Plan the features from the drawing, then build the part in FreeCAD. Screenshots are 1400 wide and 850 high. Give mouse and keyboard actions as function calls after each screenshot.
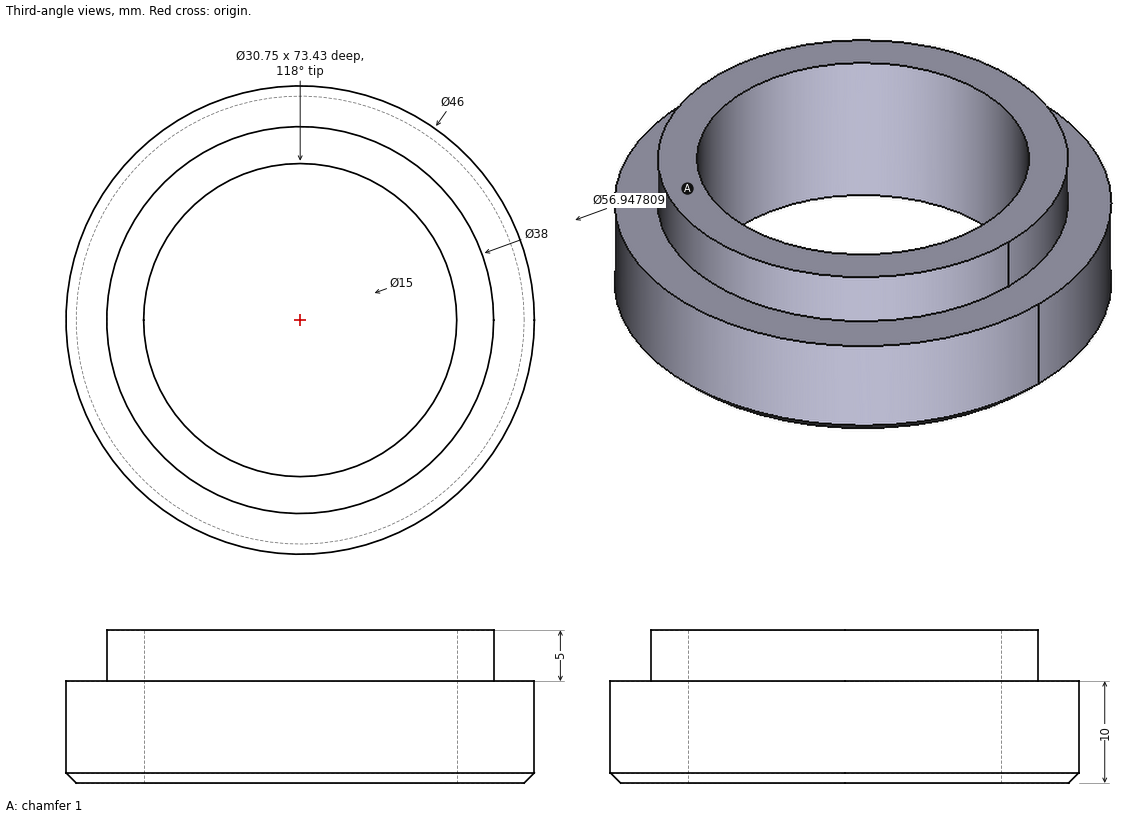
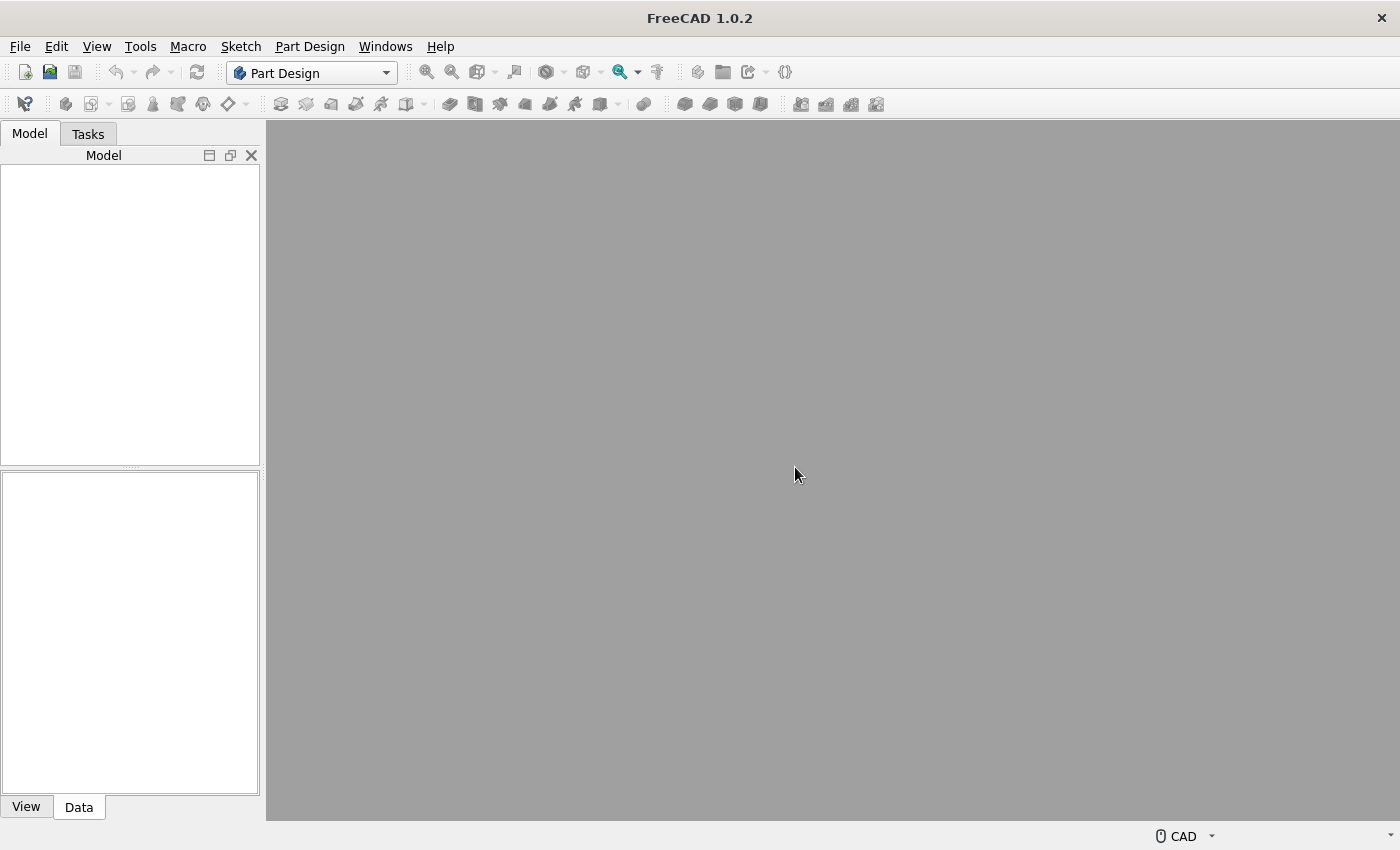
click(25, 72)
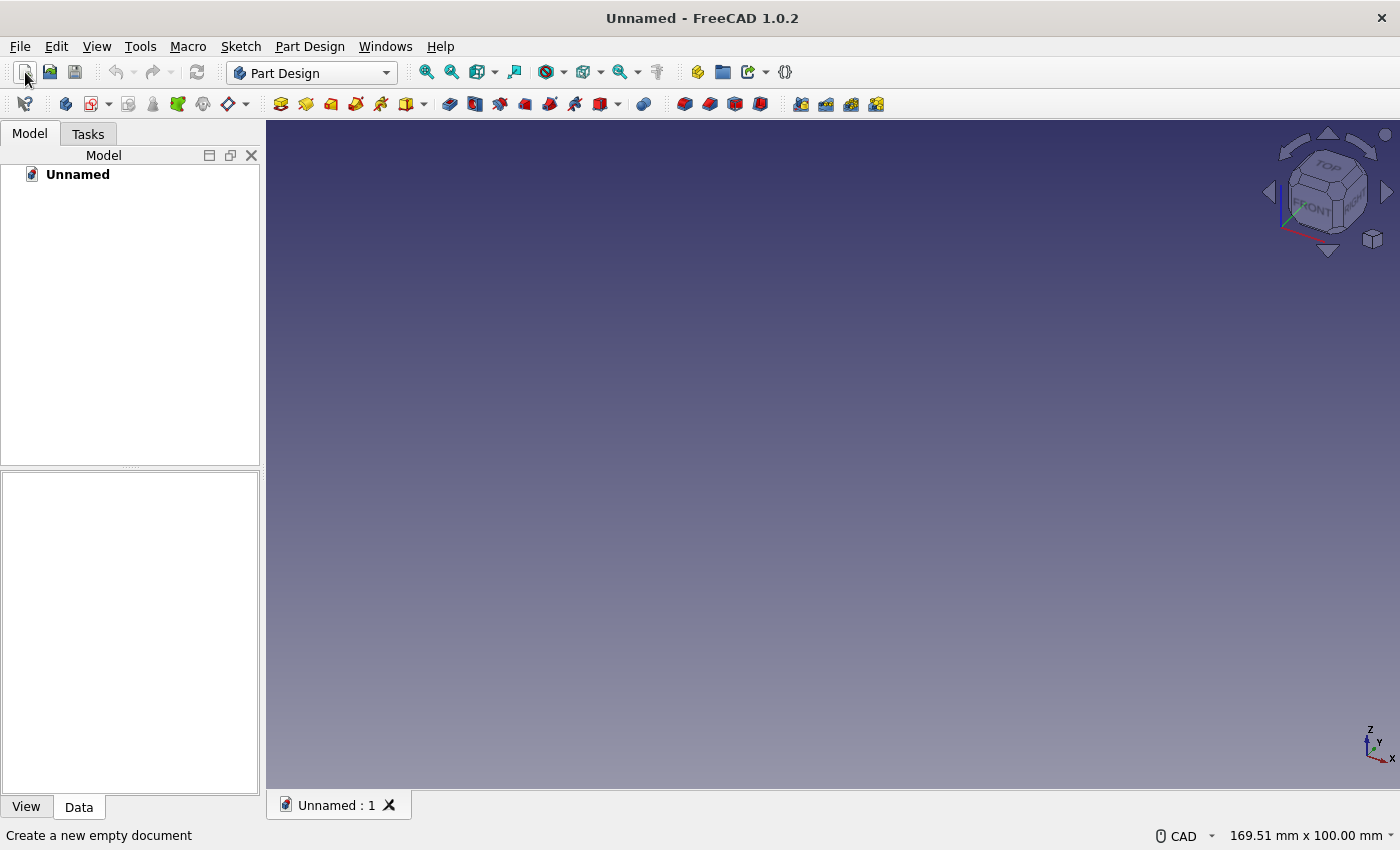
click(90, 104)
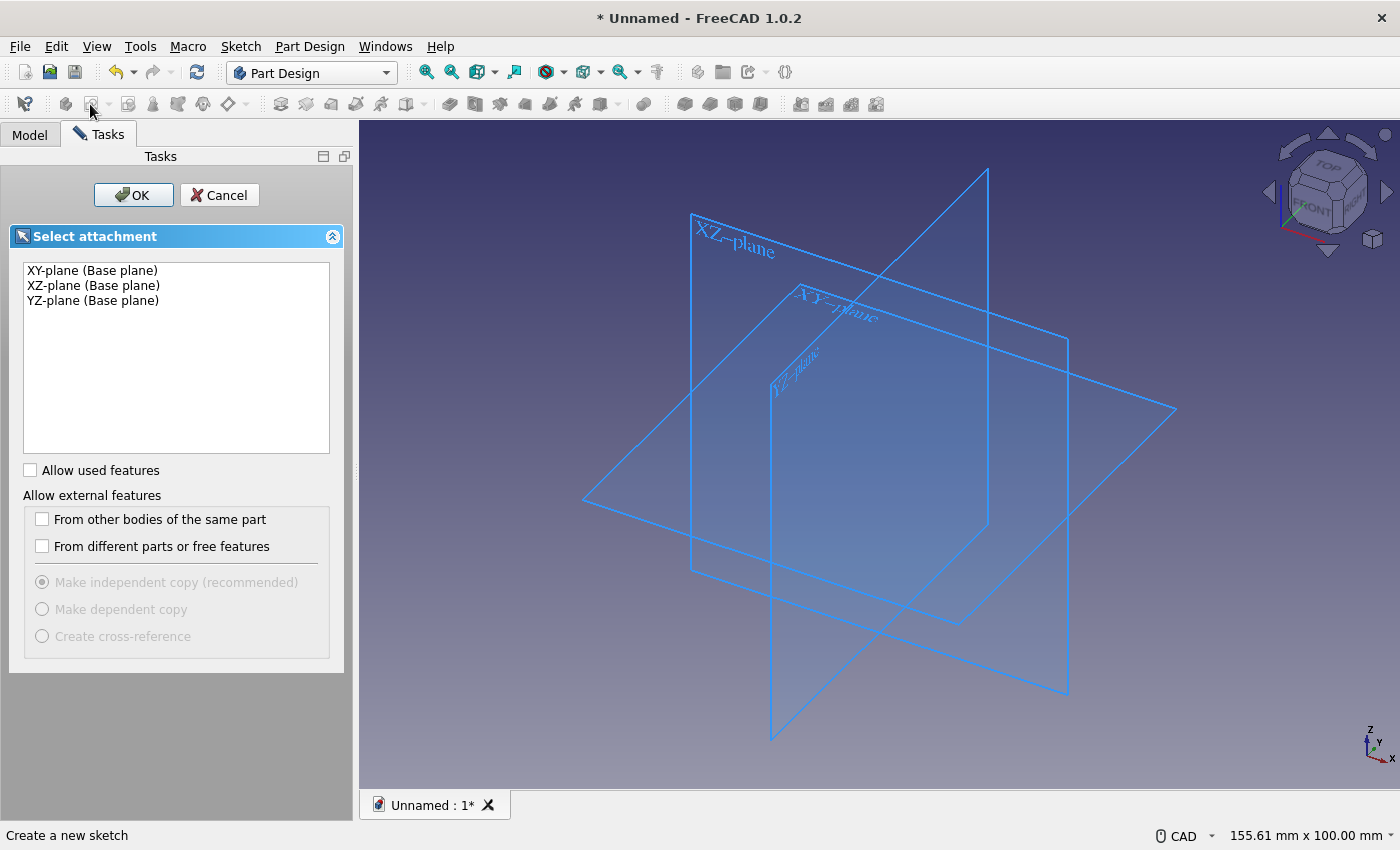
click(84, 270)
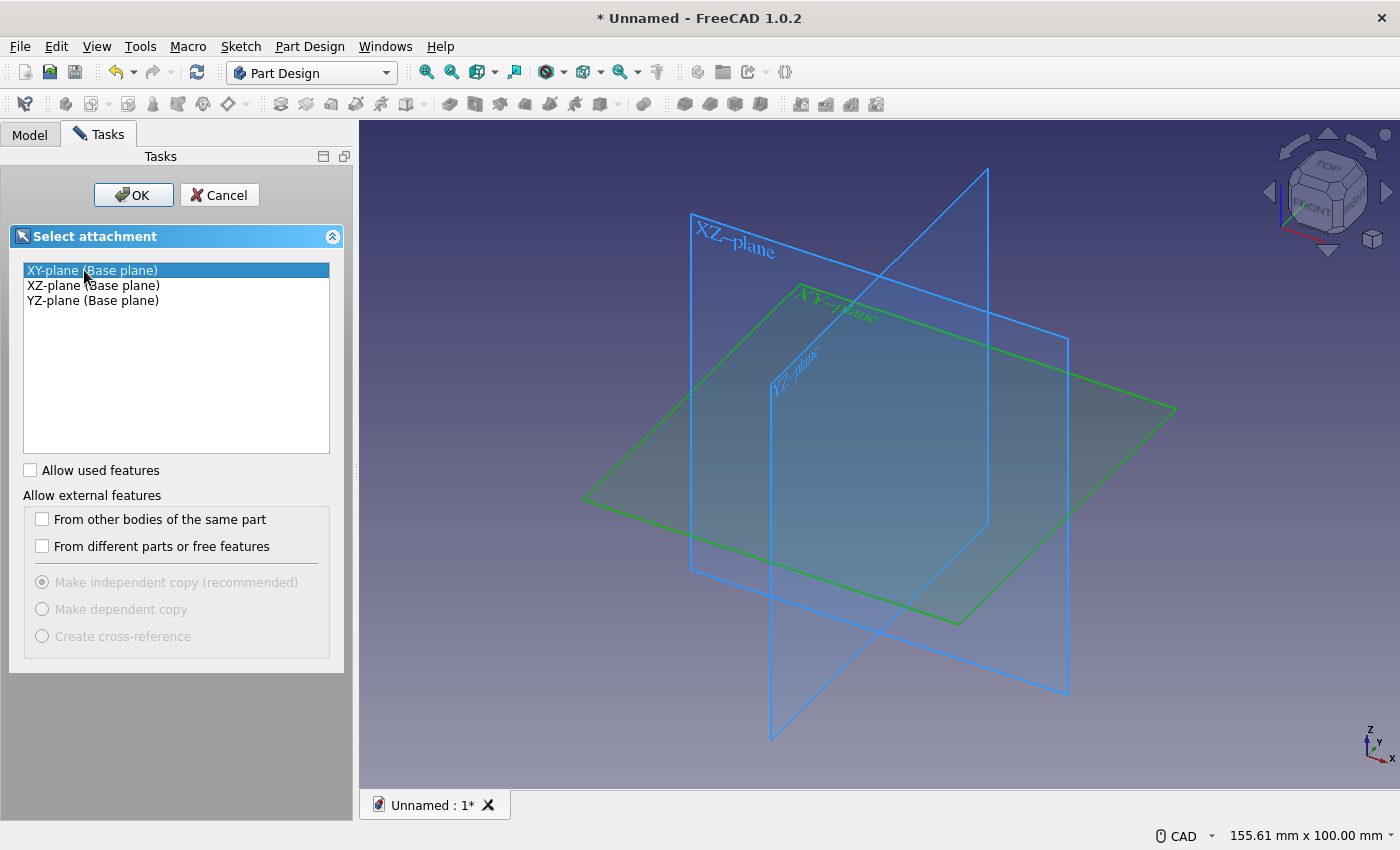
click(134, 195)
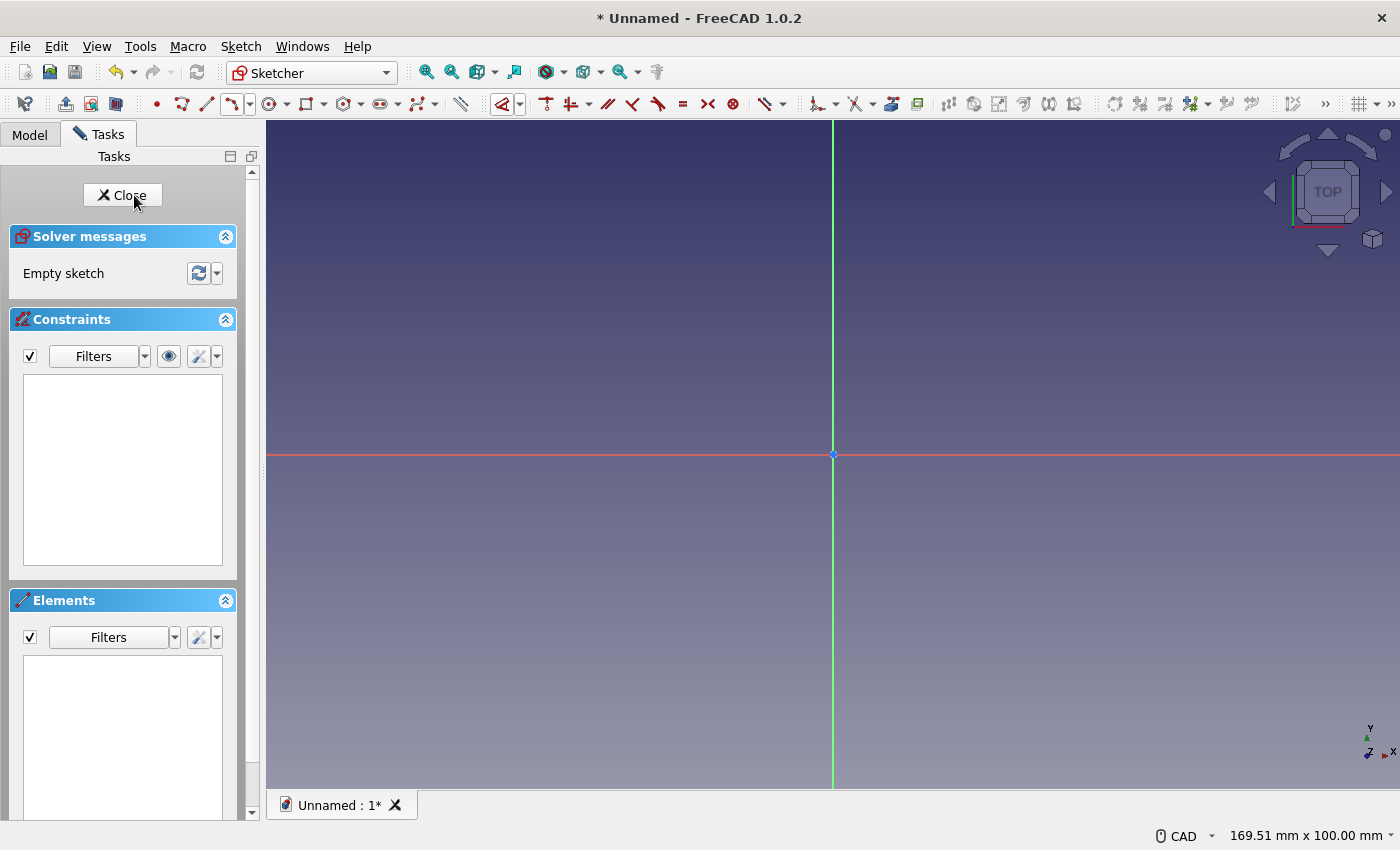
scroll(916, 454, up, 3)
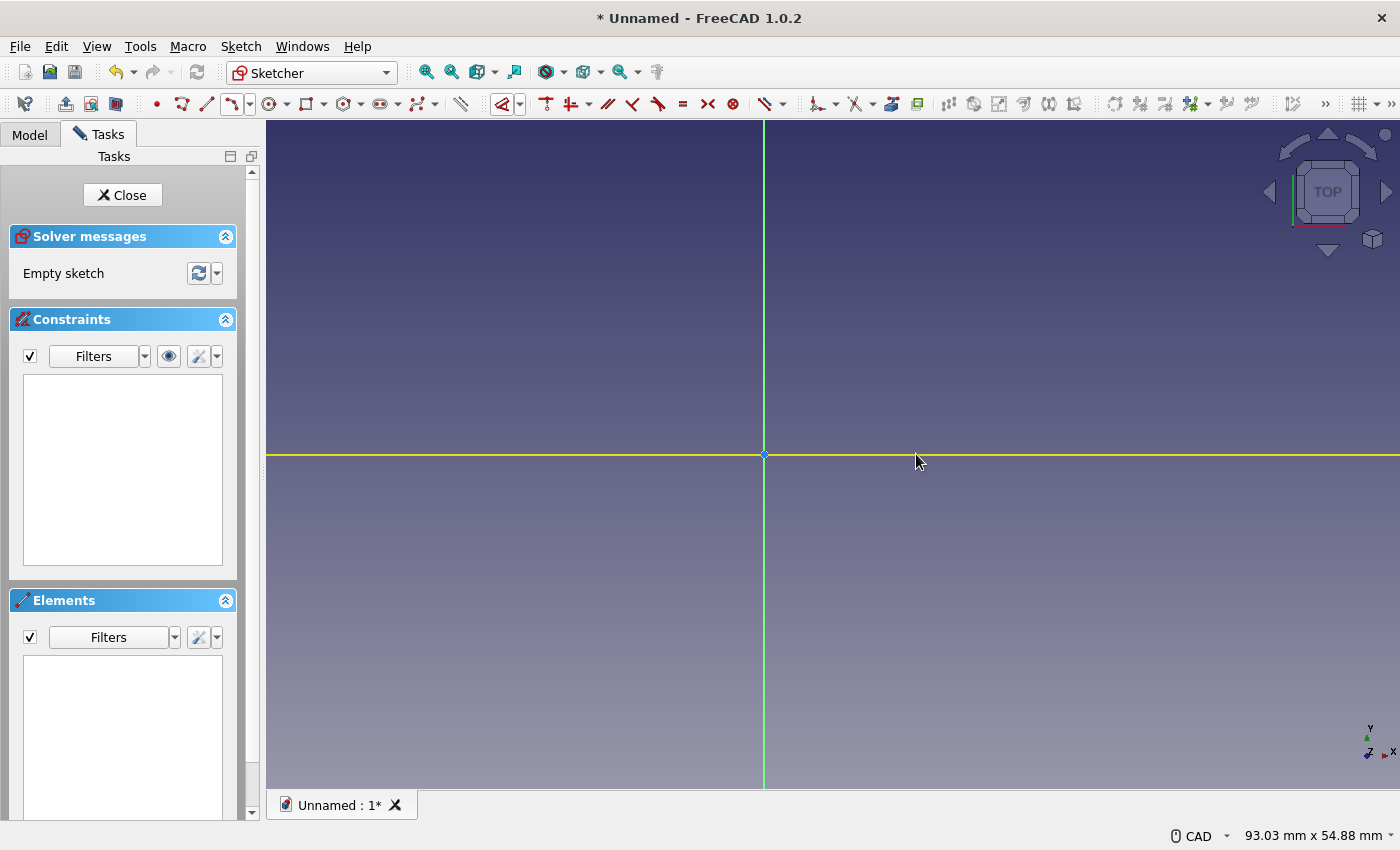
click(268, 104)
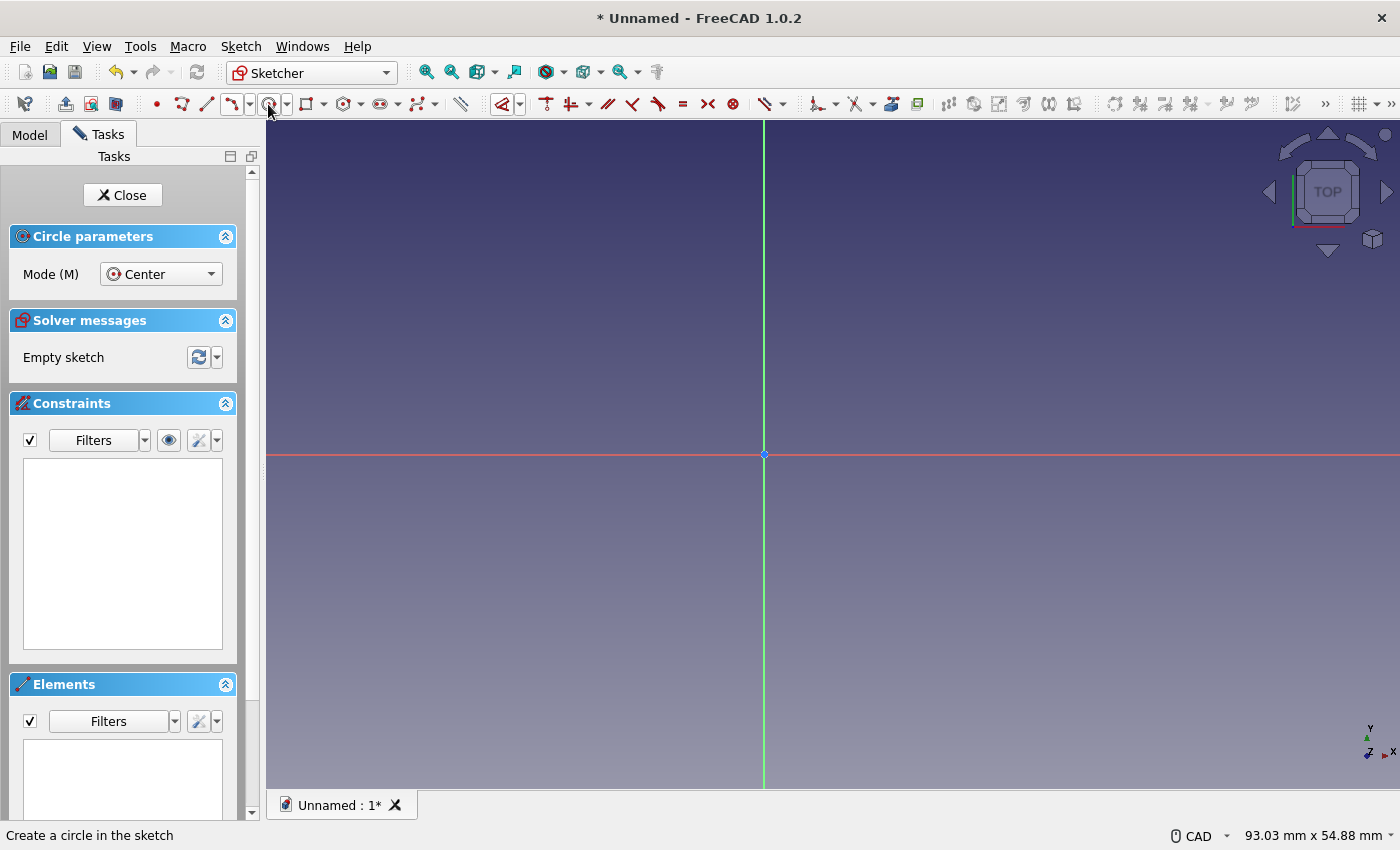
click(764, 454)
move(928, 291)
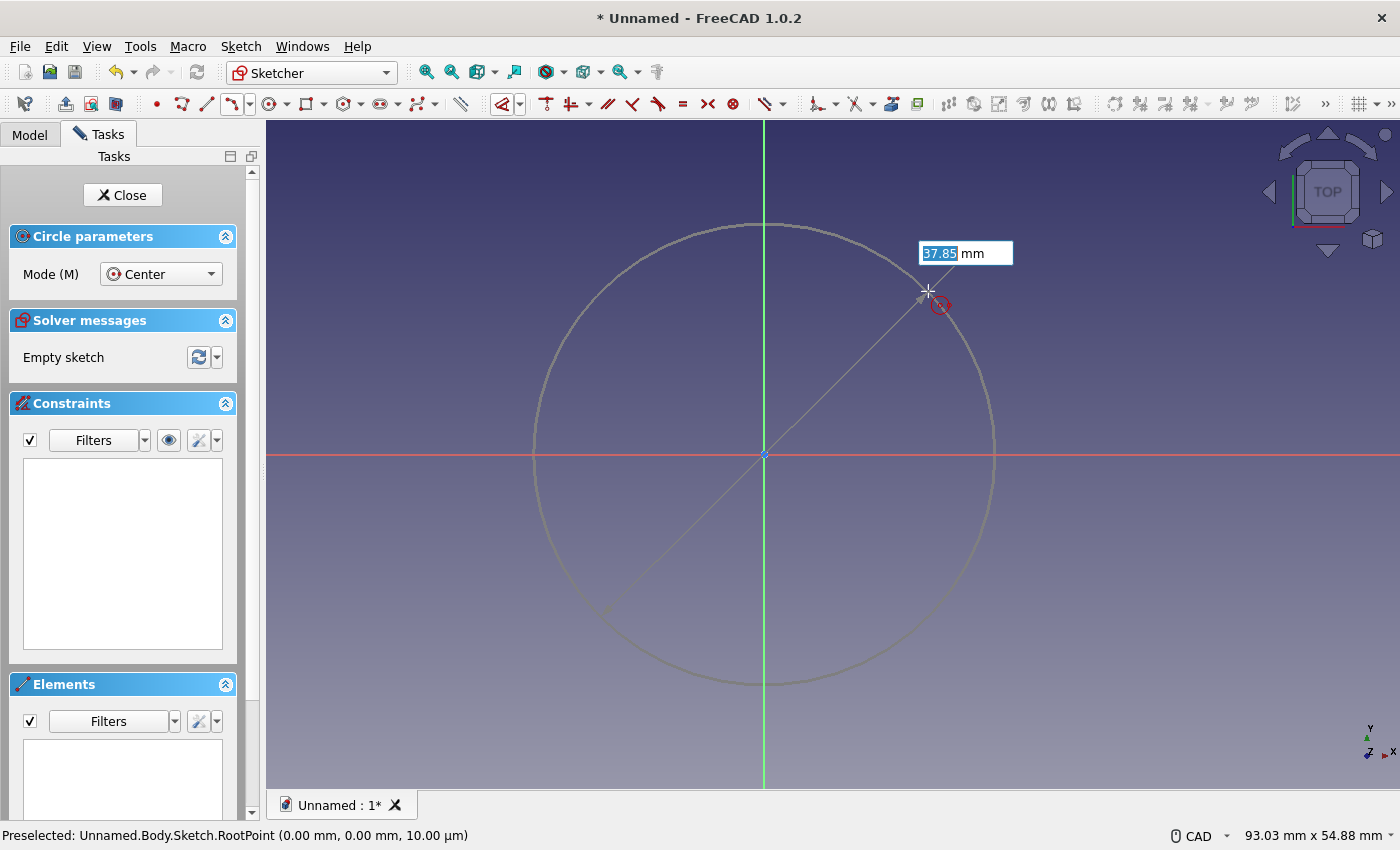
text(38)
key(Return)